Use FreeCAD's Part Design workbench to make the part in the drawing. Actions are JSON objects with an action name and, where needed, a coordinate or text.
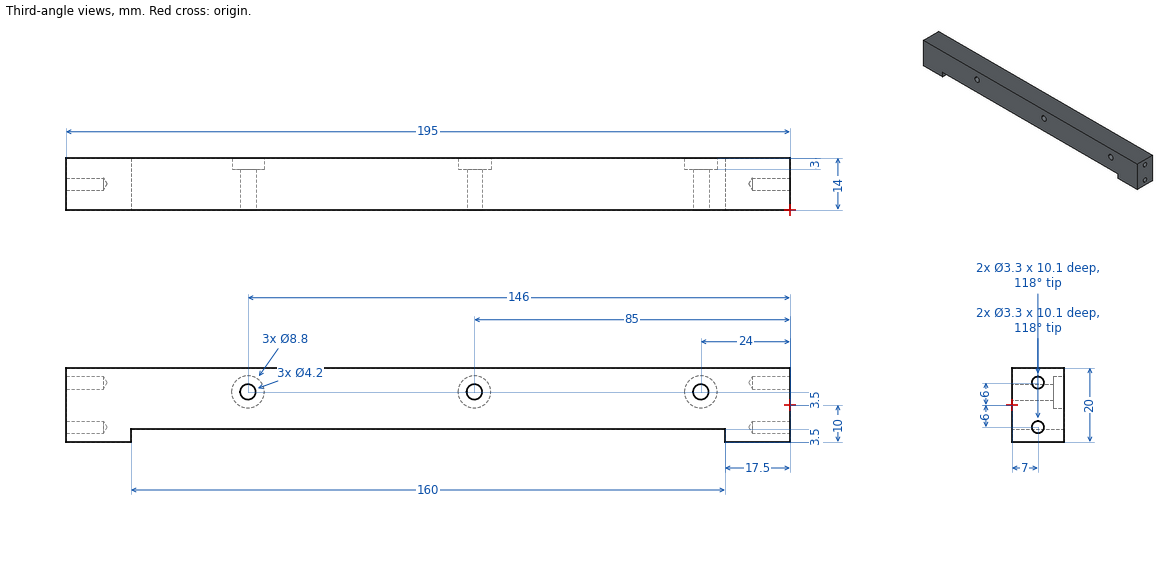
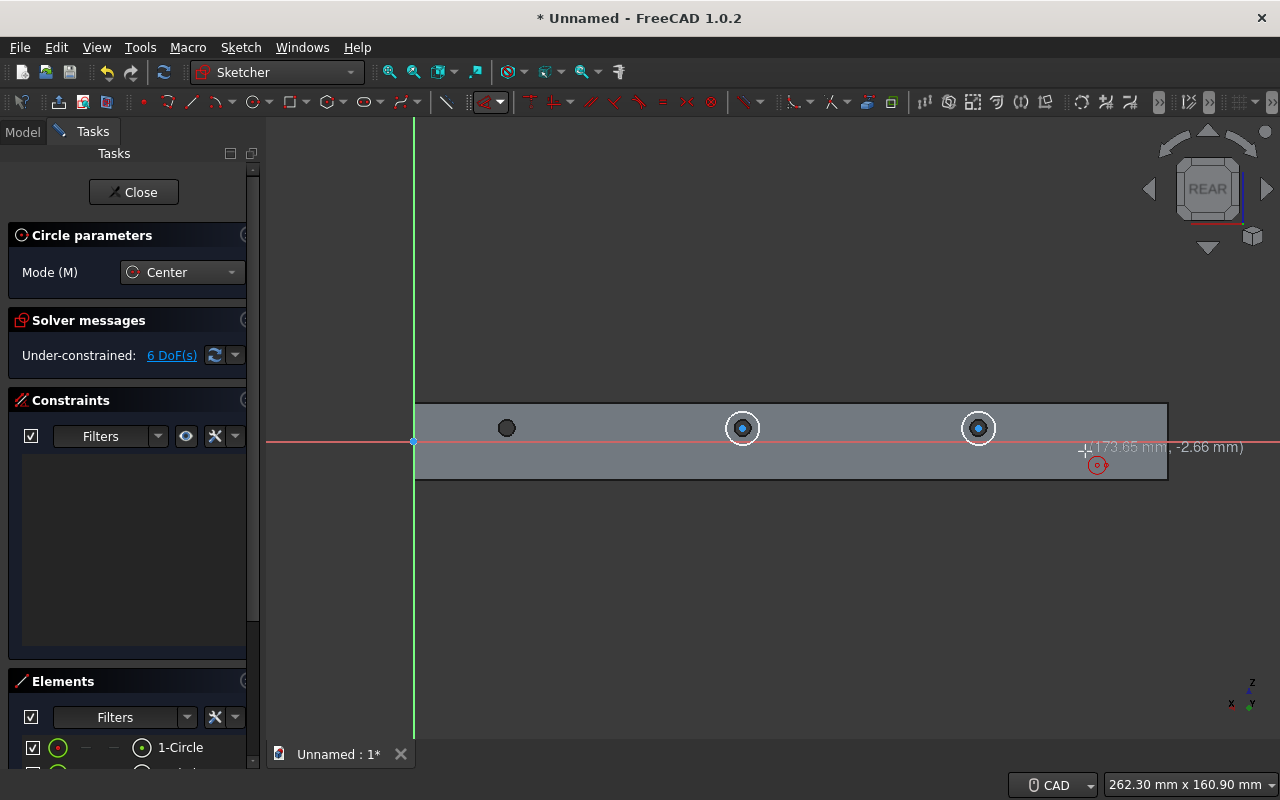
{"action": "scroll", "coordinate": [507, 428], "scroll_direction": "up", "scroll_amount": 2}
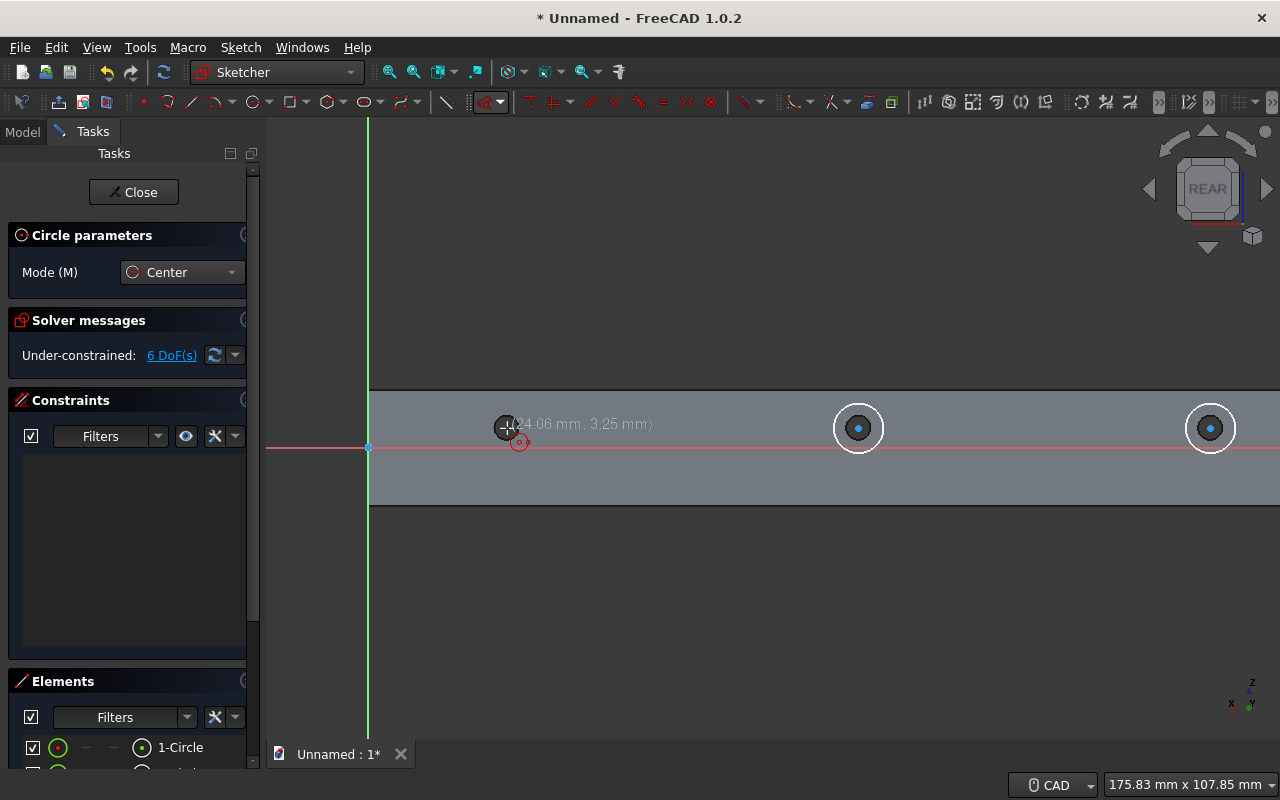
{"action": "left_click", "coordinate": [507, 428]}
{"action": "left_click", "coordinate": [524, 410]}
{"action": "key", "text": "Escape"}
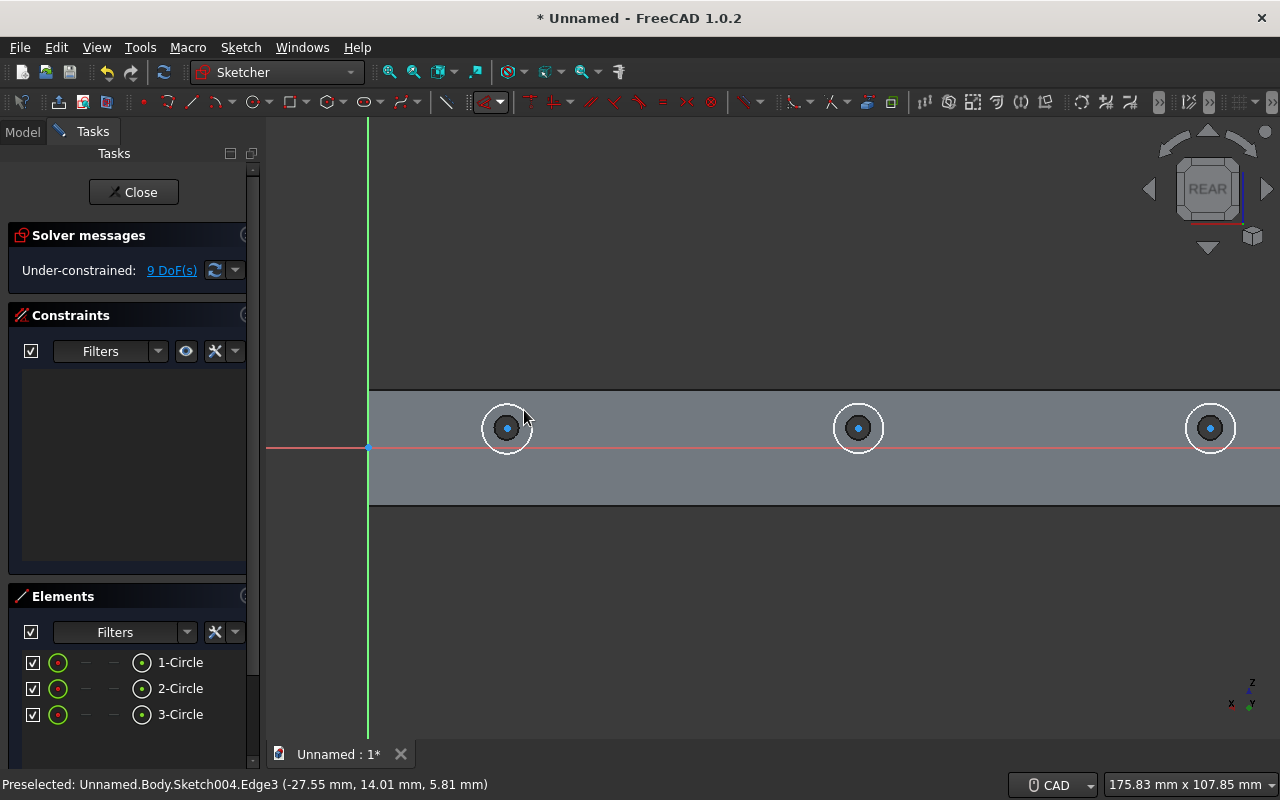
{"action": "scroll", "coordinate": [507, 428], "scroll_direction": "down", "scroll_amount": 2}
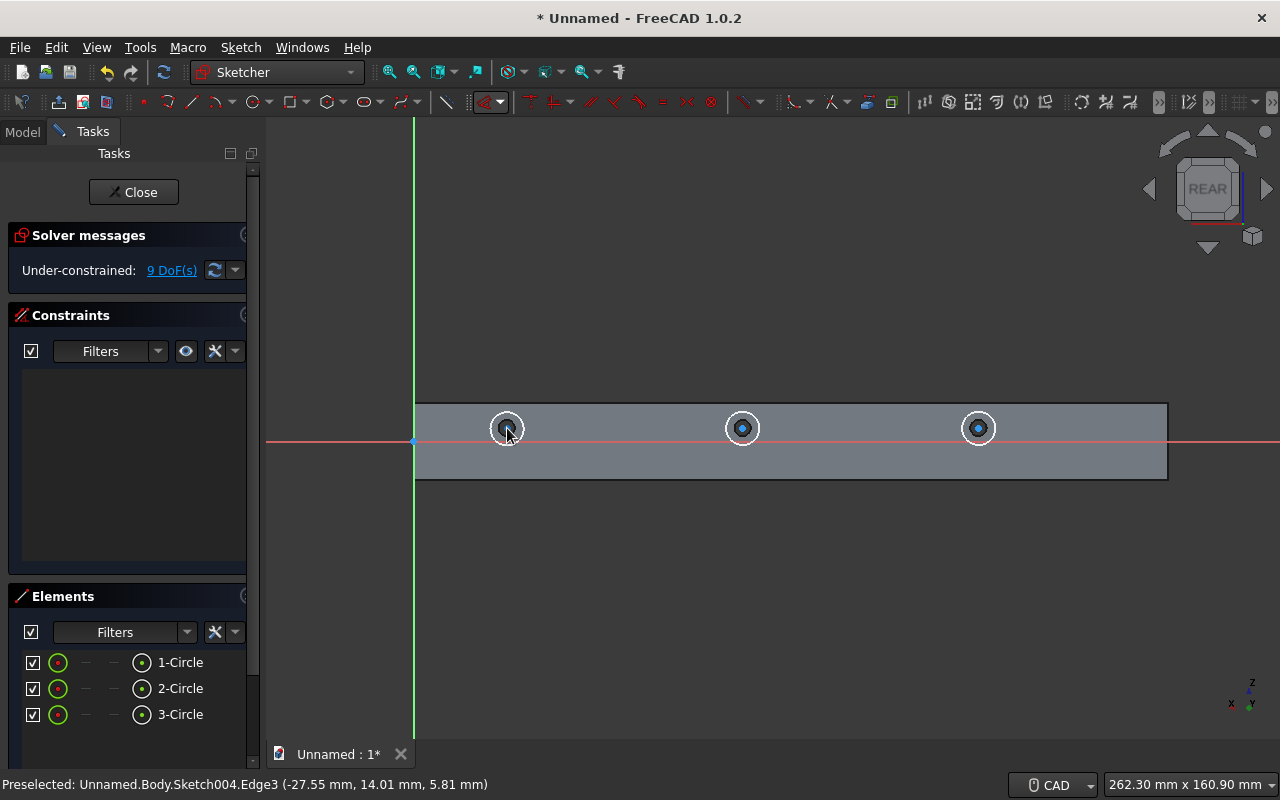
{"action": "left_click", "coordinate": [990, 417]}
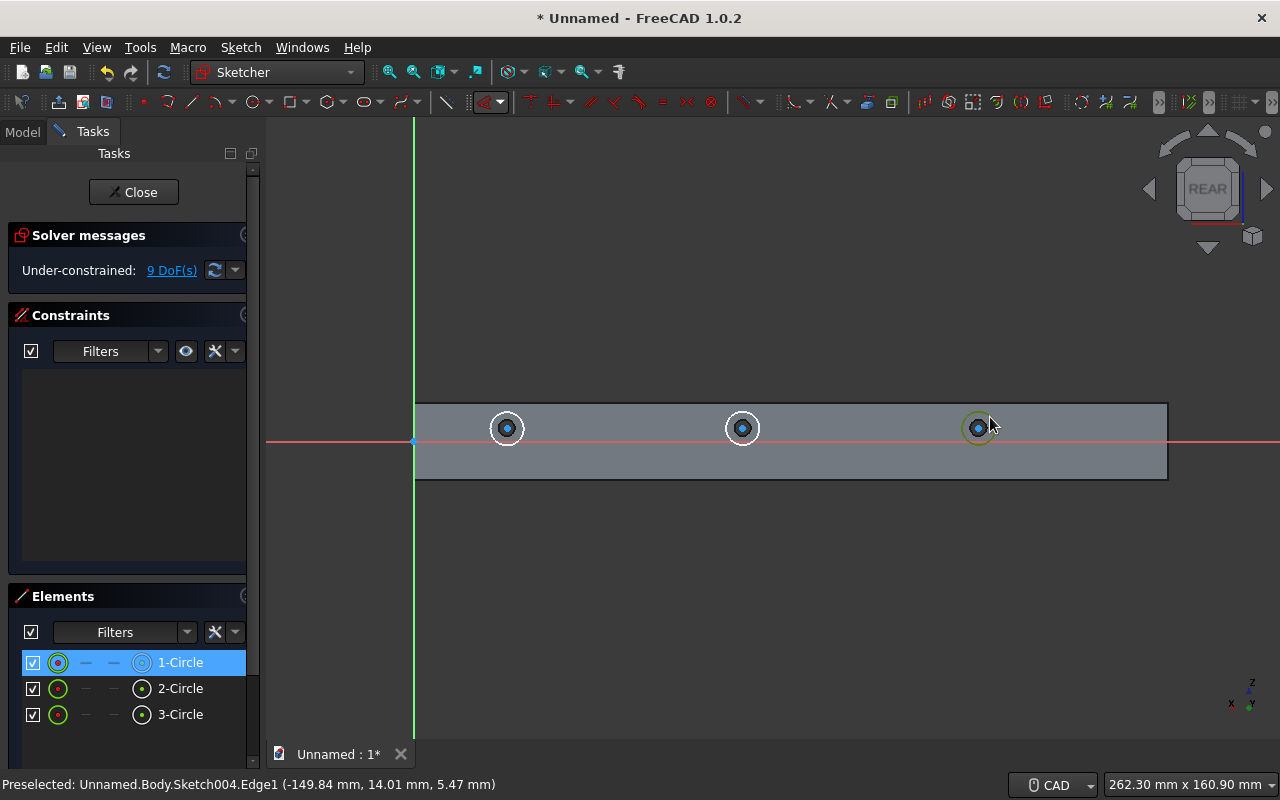
{"action": "left_click", "coordinate": [754, 417]}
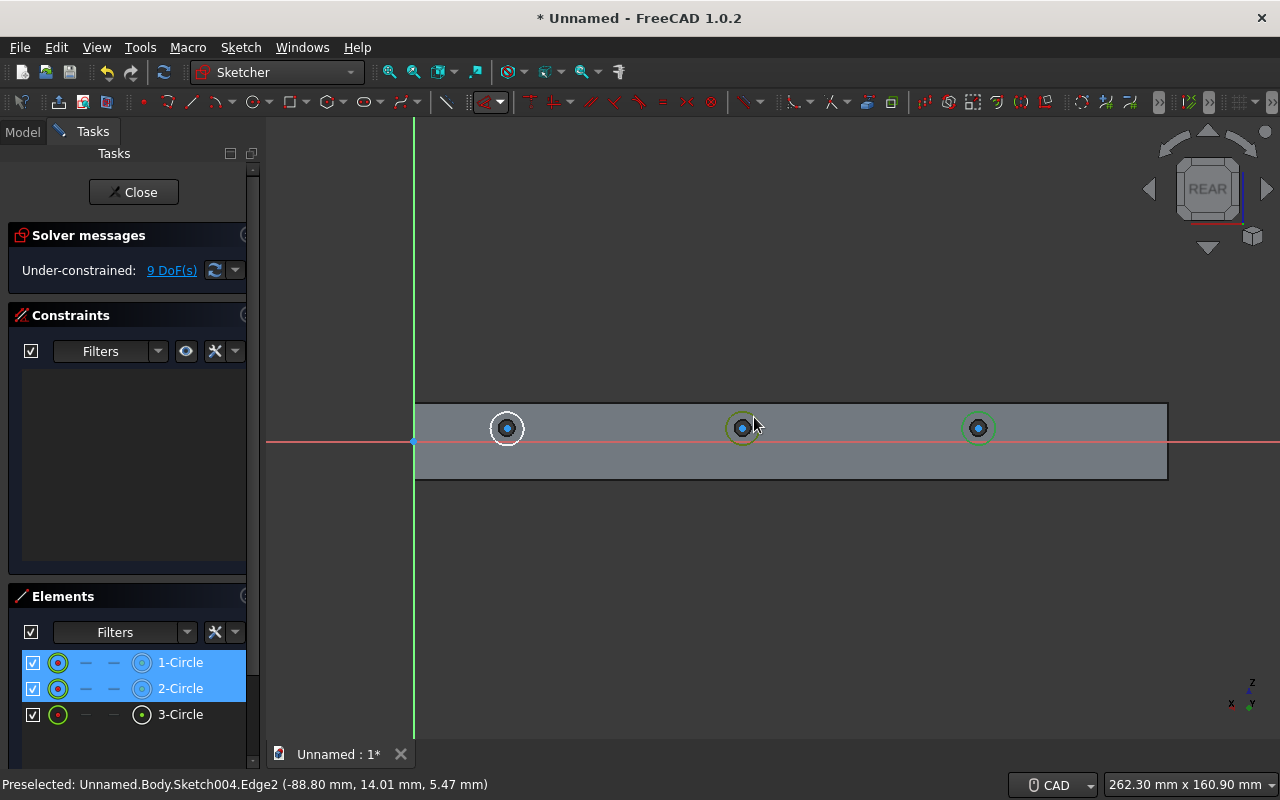
{"action": "left_click", "coordinate": [519, 417]}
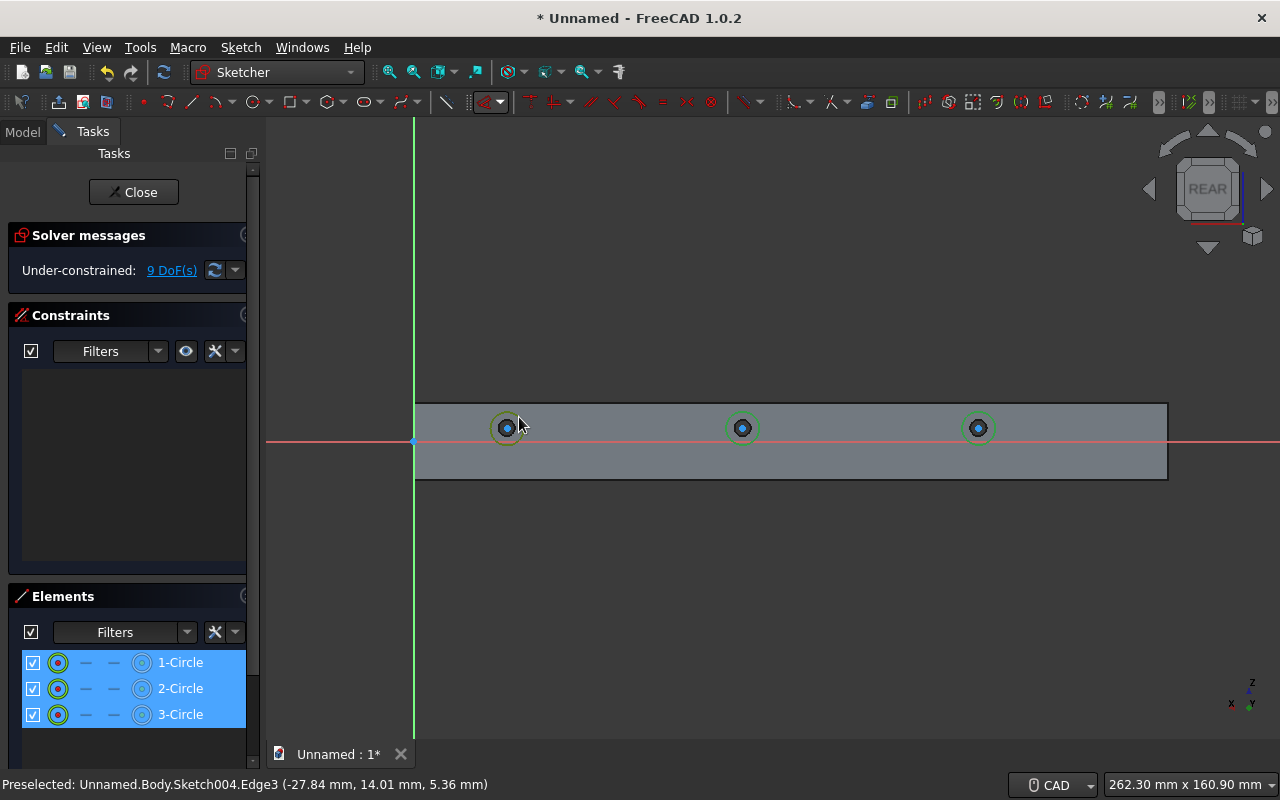
{"action": "key", "text": "e"}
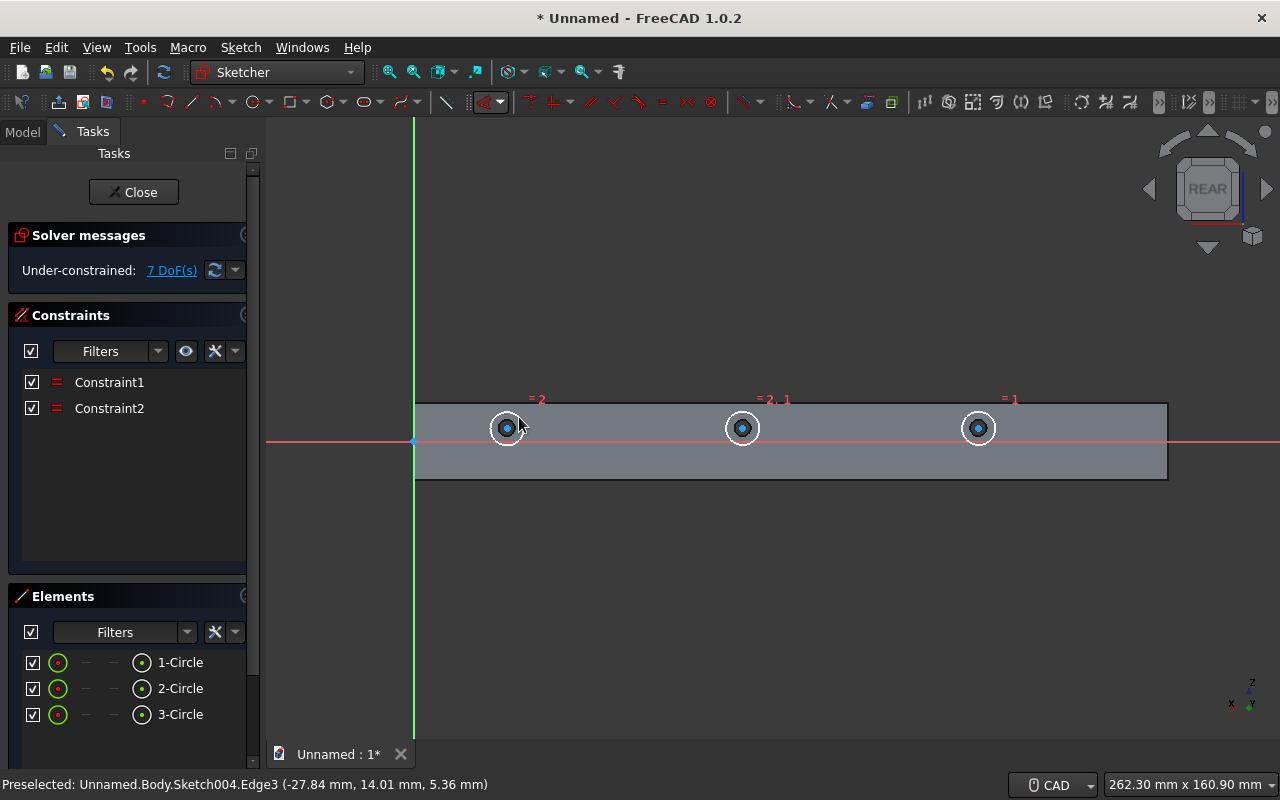
{"action": "left_click", "coordinate": [990, 417]}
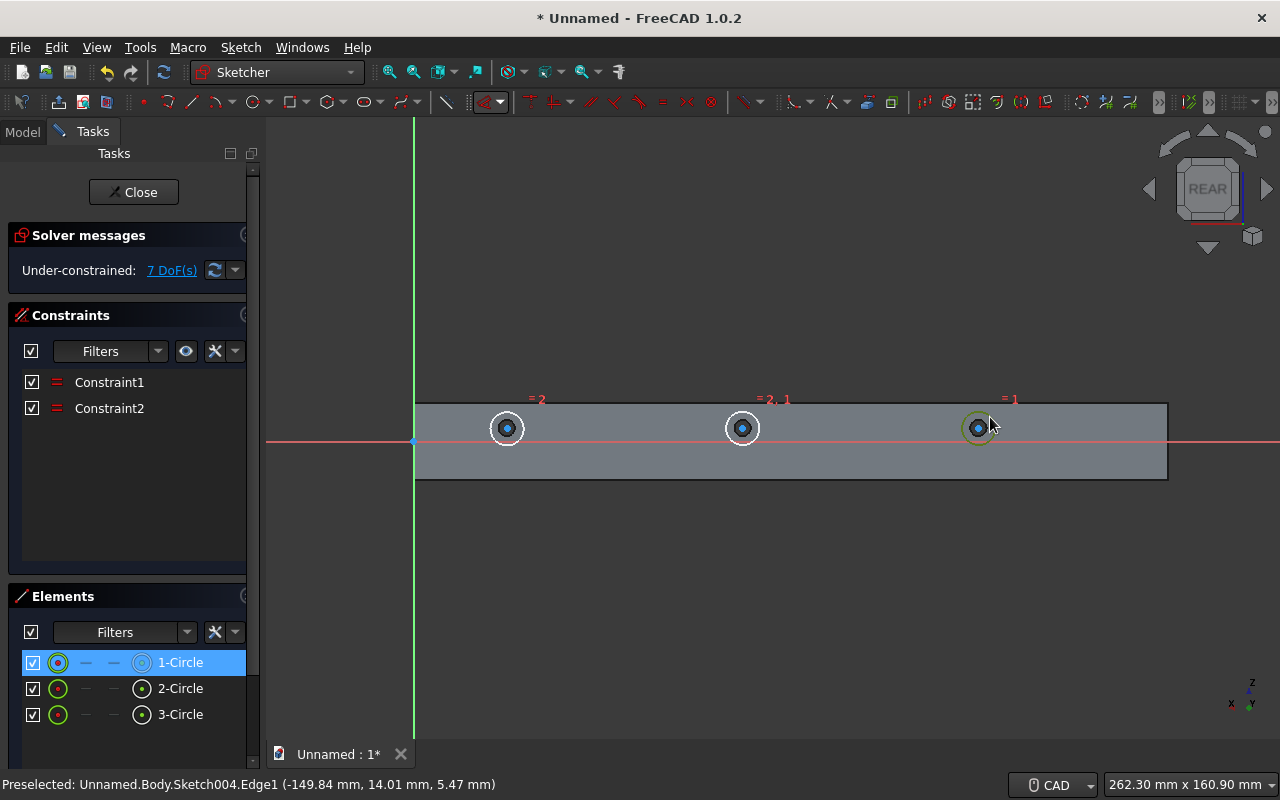
{"action": "key", "text": "k o"}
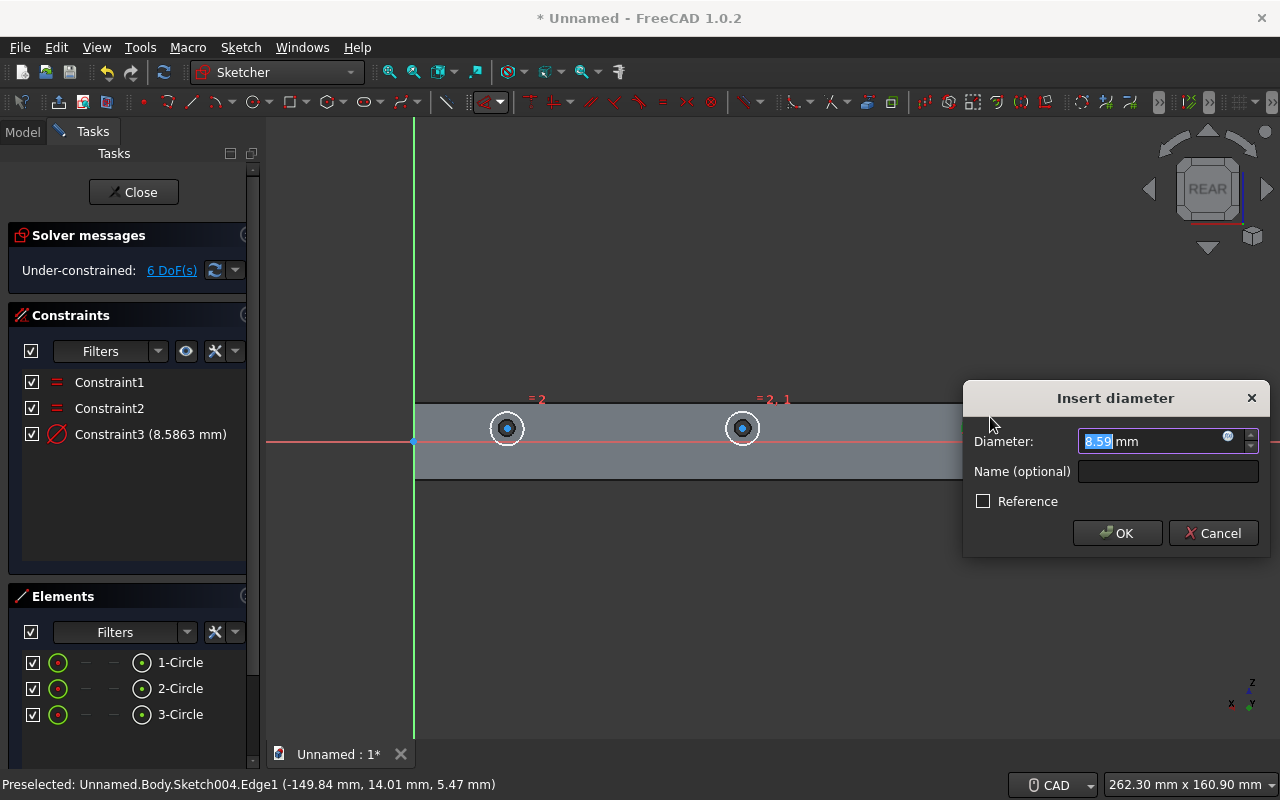
{"action": "type", "text": "8.8"}
{"action": "key", "text": "Return"}